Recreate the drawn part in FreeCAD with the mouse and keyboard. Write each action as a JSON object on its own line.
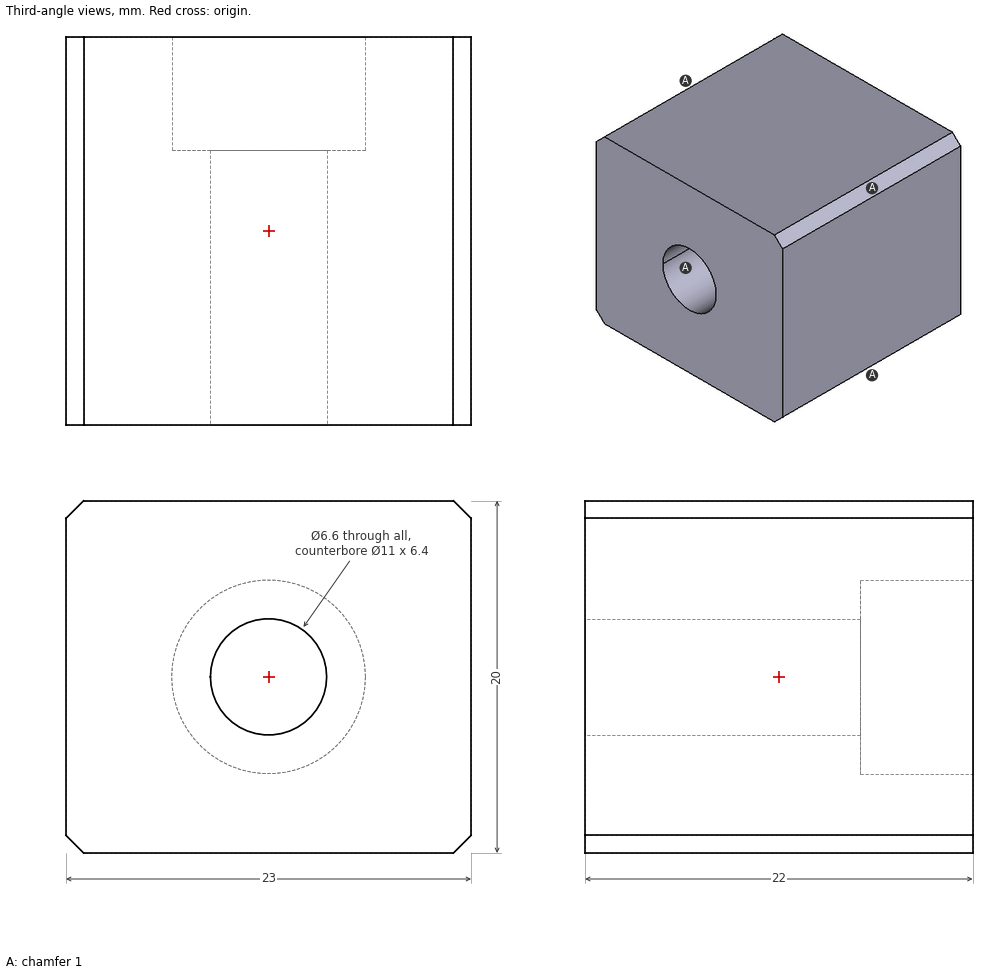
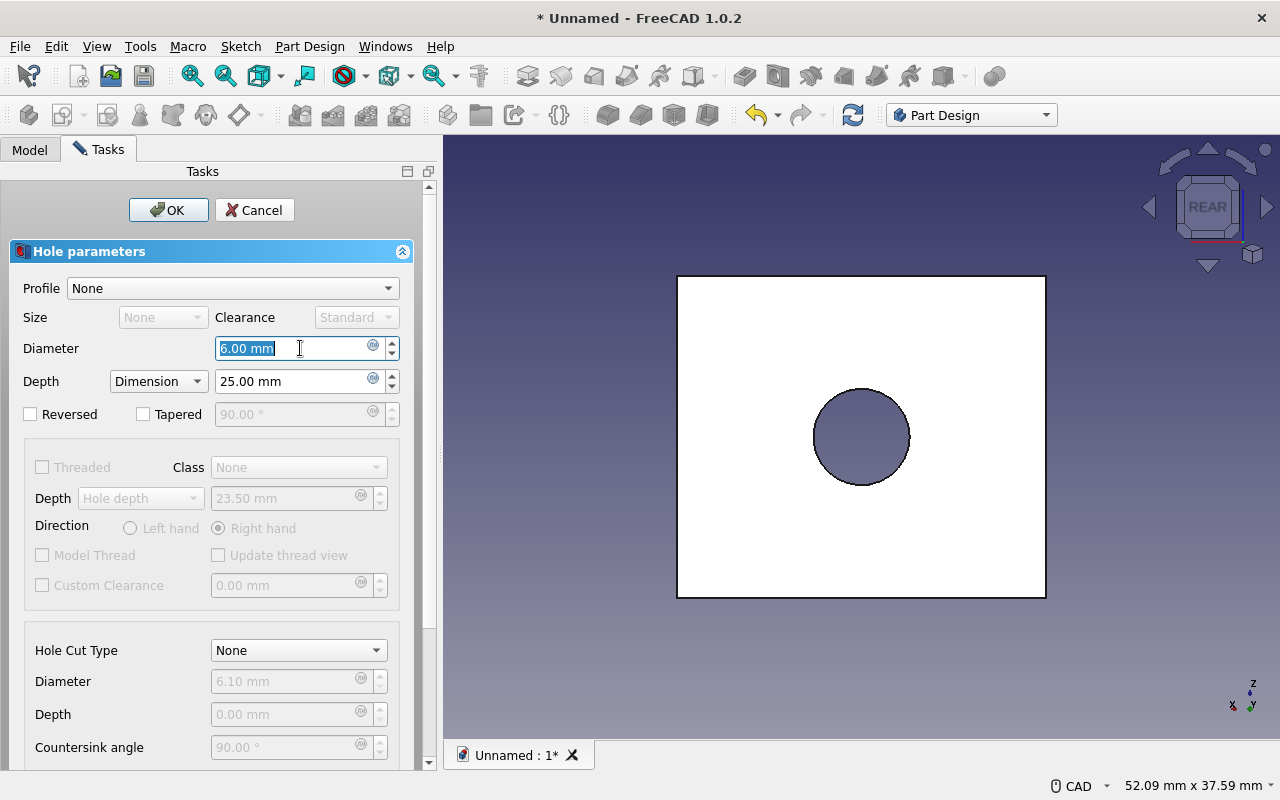
{"action": "type", "text": "6.6"}
{"action": "key", "text": "Tab"}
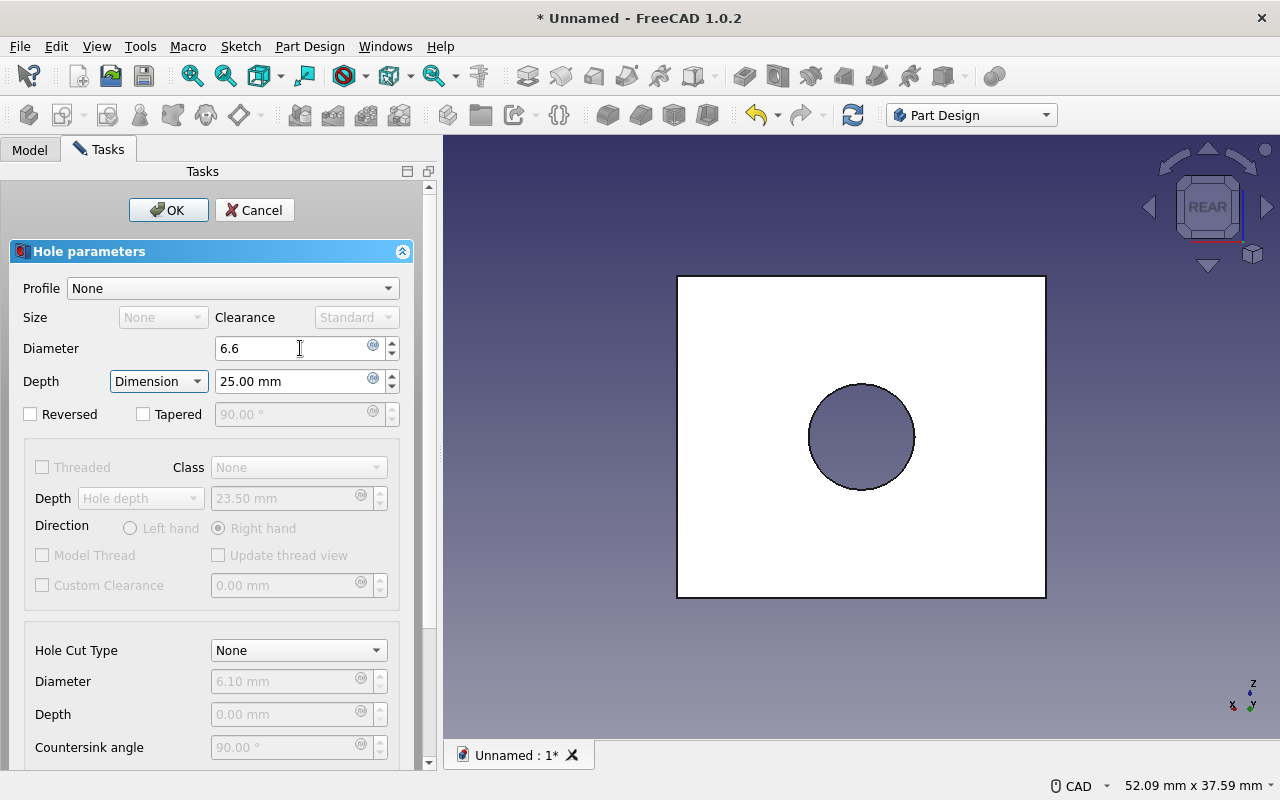
{"action": "left_click", "coordinate": [160, 382]}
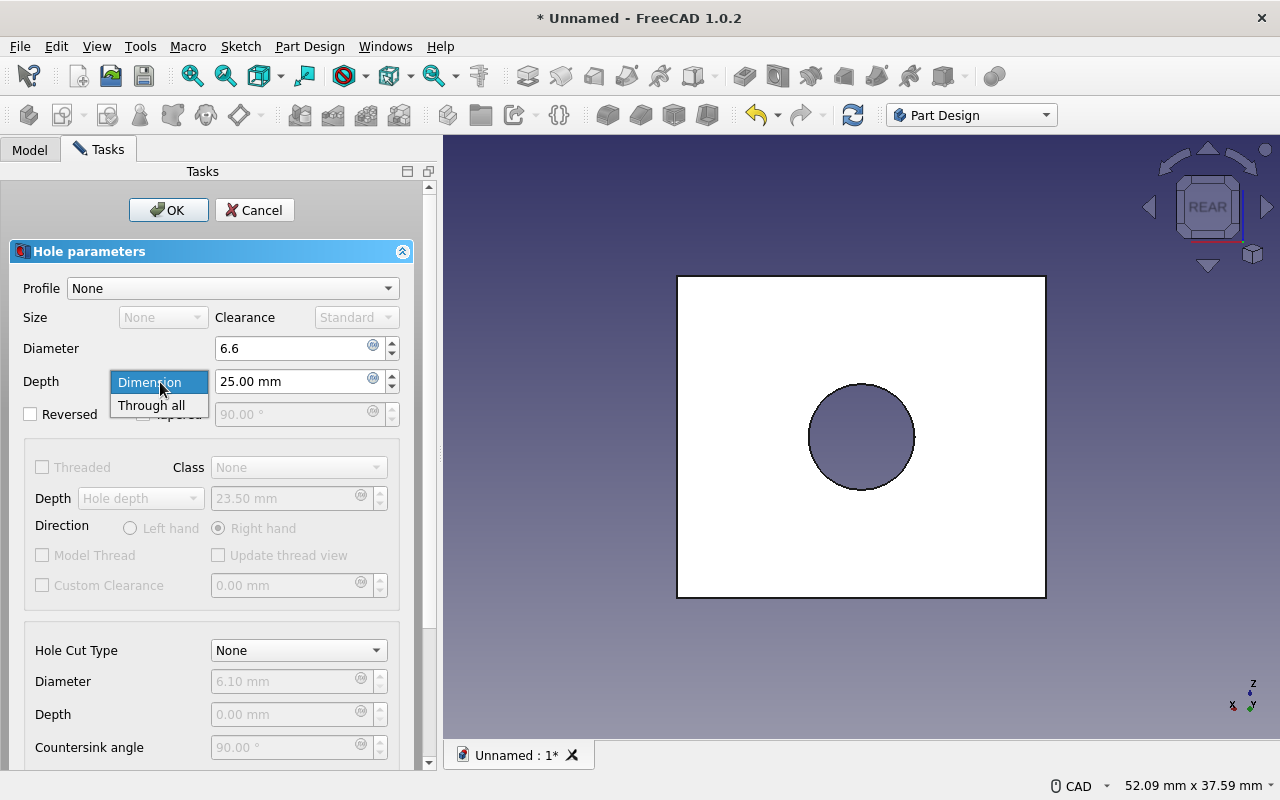
{"action": "left_click", "coordinate": [158, 406]}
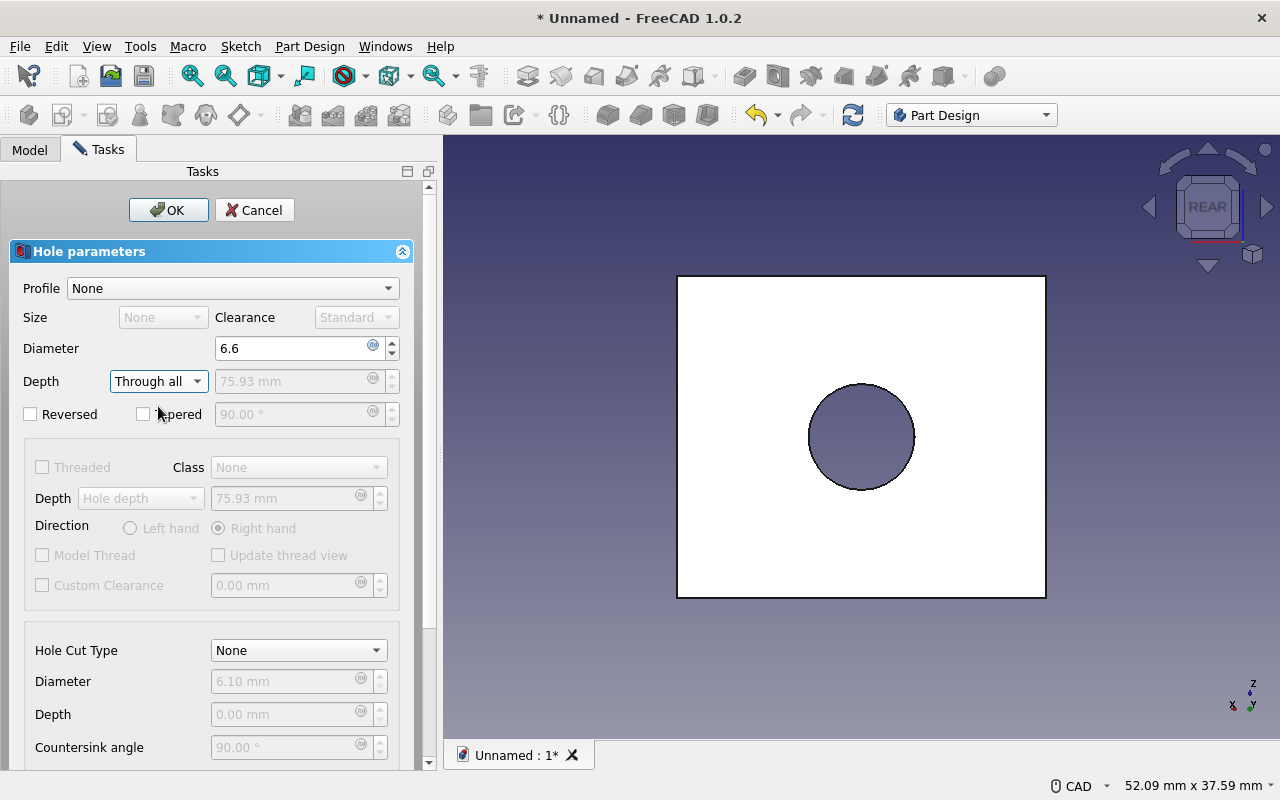
{"action": "left_click", "coordinate": [300, 650]}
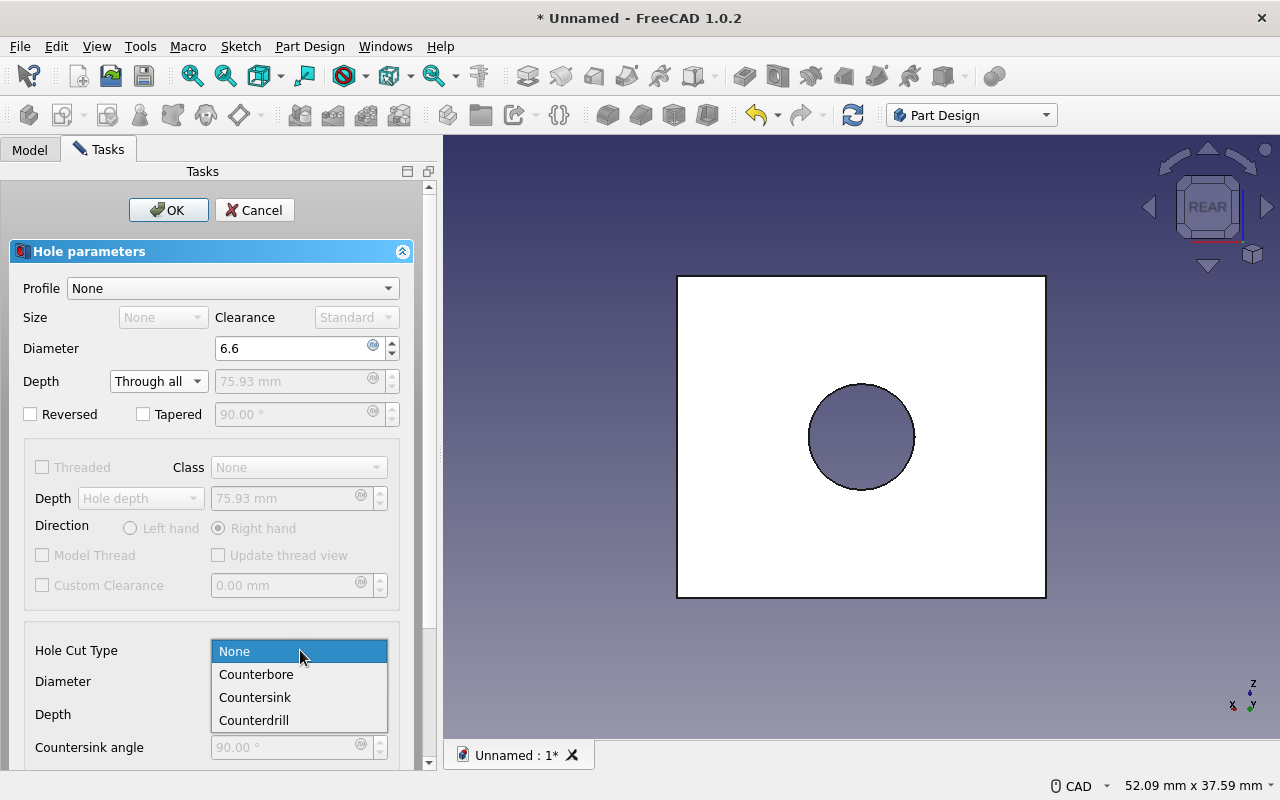
{"action": "left_click", "coordinate": [298, 674]}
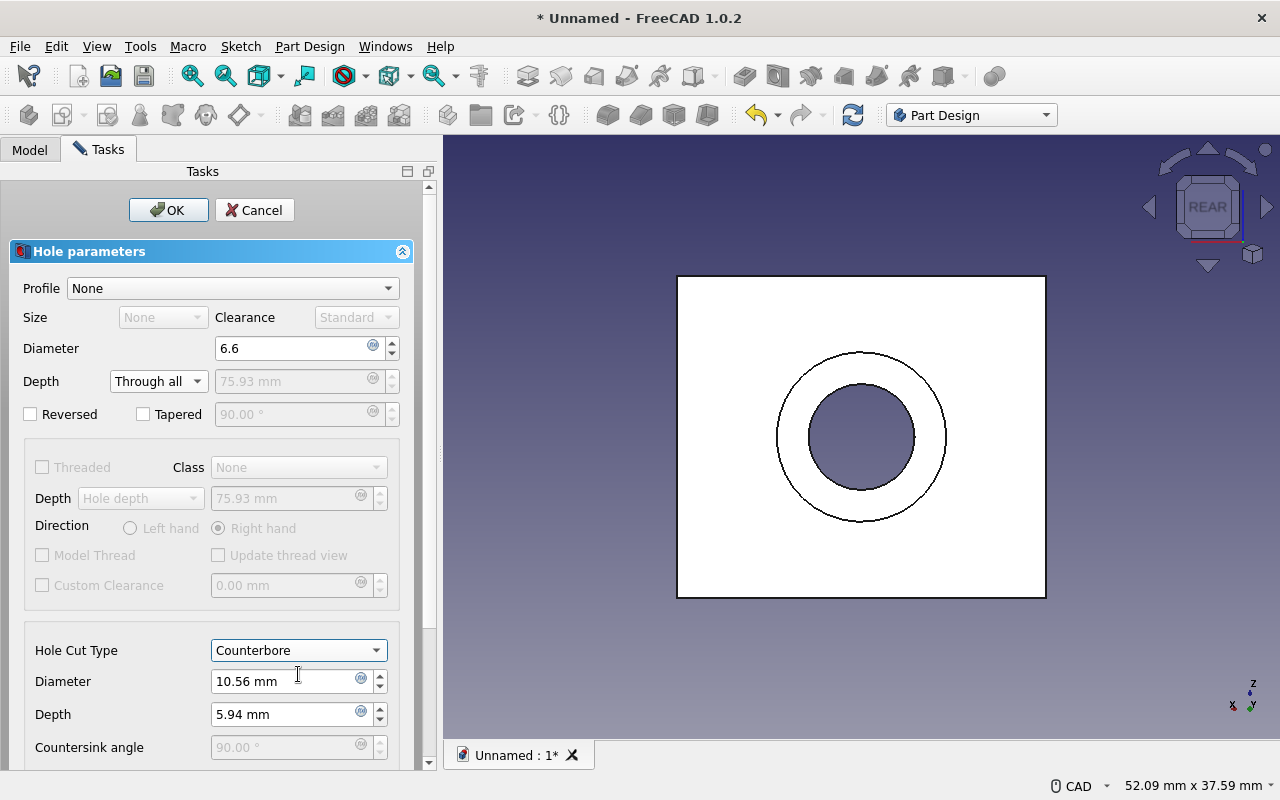
{"action": "triple_click", "coordinate": [292, 682]}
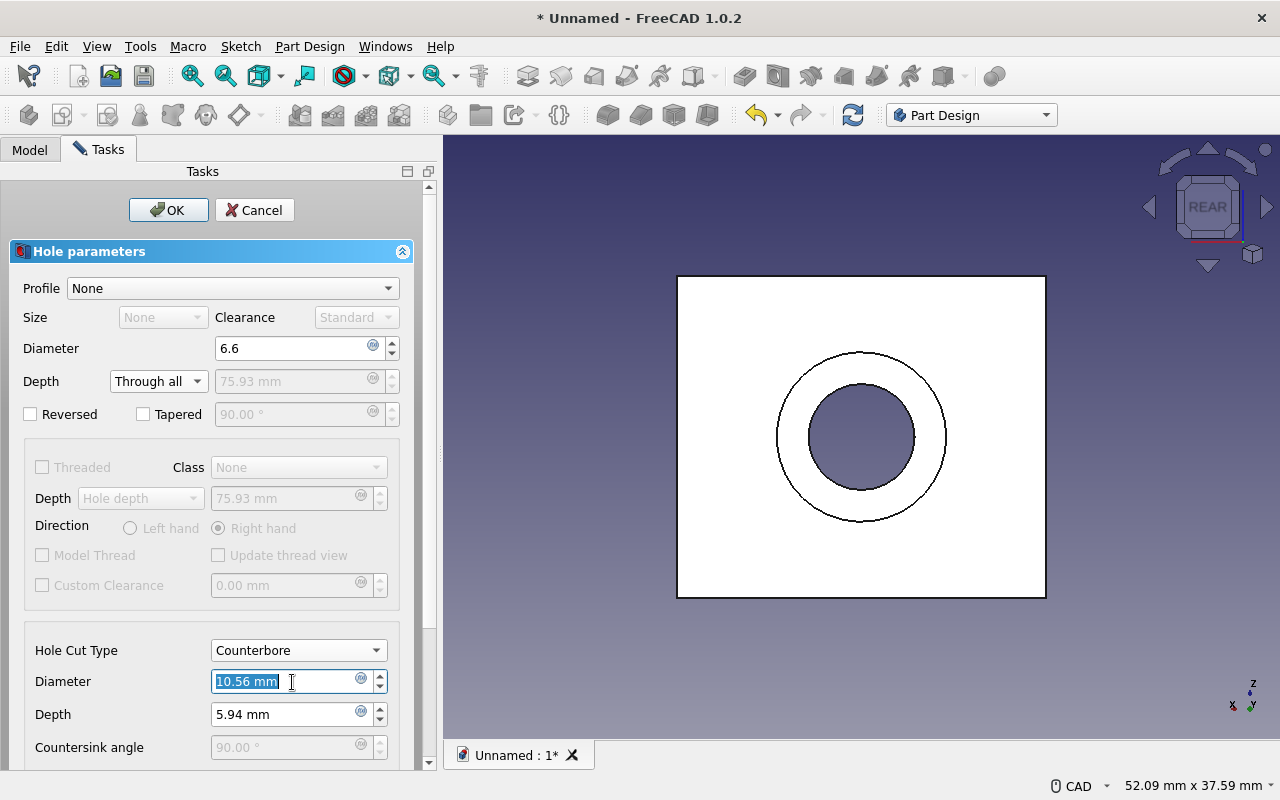
{"action": "type", "text": "11"}
{"action": "key", "text": "Tab"}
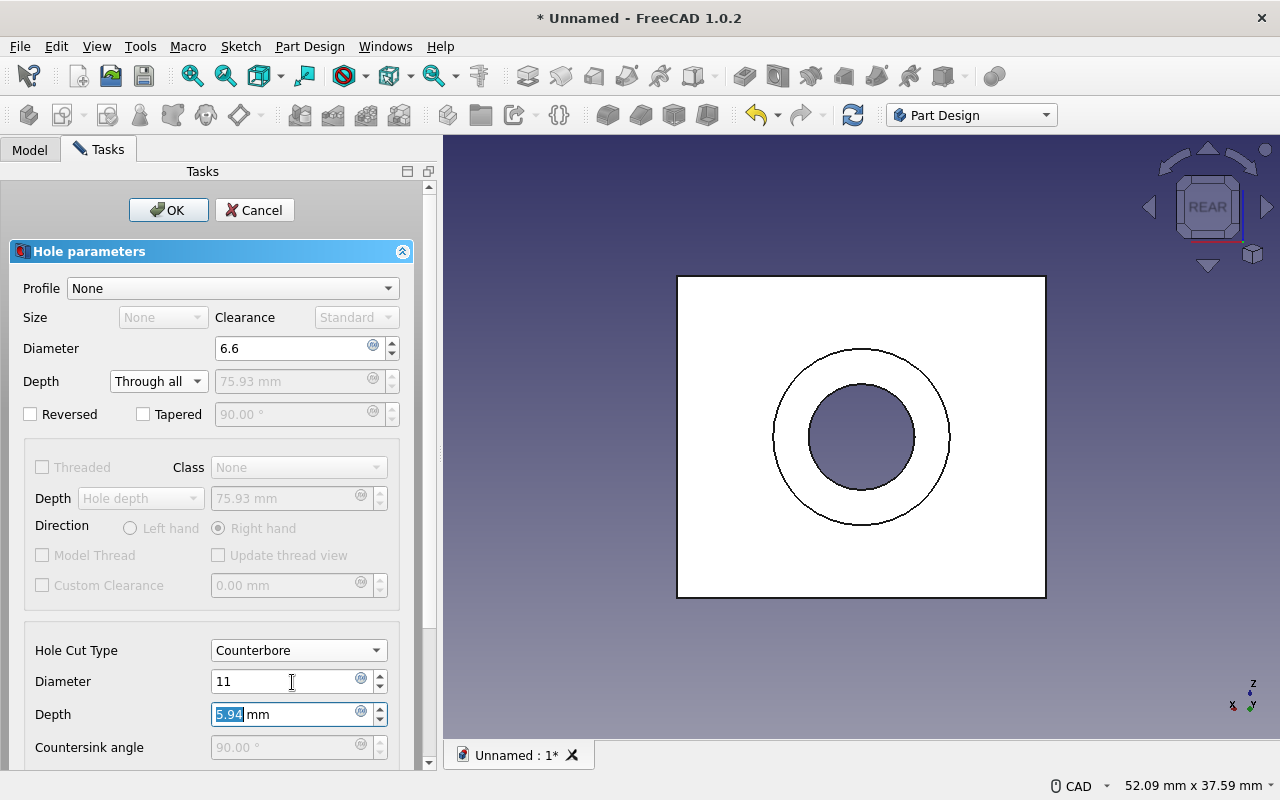
{"action": "type", "text": "6.4"}
{"action": "key", "text": "Tab"}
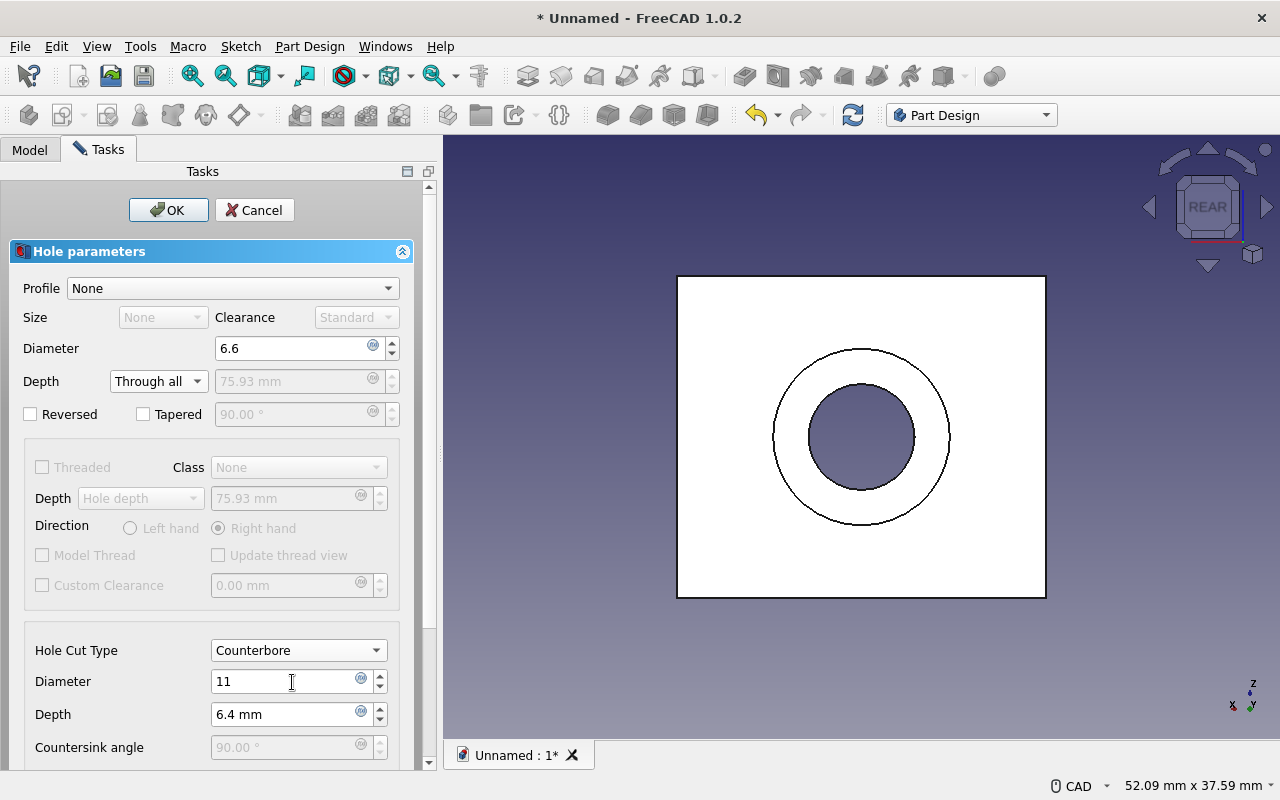
{"action": "left_click", "coordinate": [169, 210]}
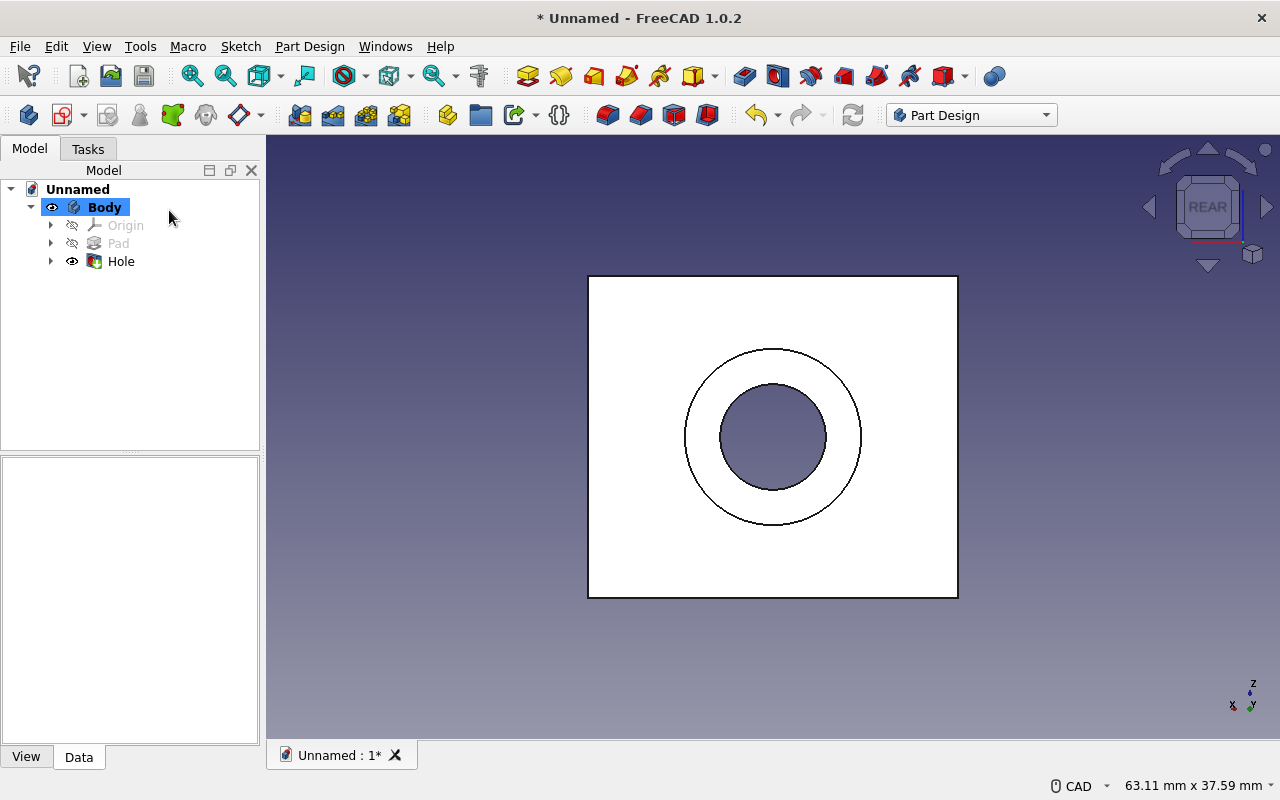
{"action": "key", "text": "0"}